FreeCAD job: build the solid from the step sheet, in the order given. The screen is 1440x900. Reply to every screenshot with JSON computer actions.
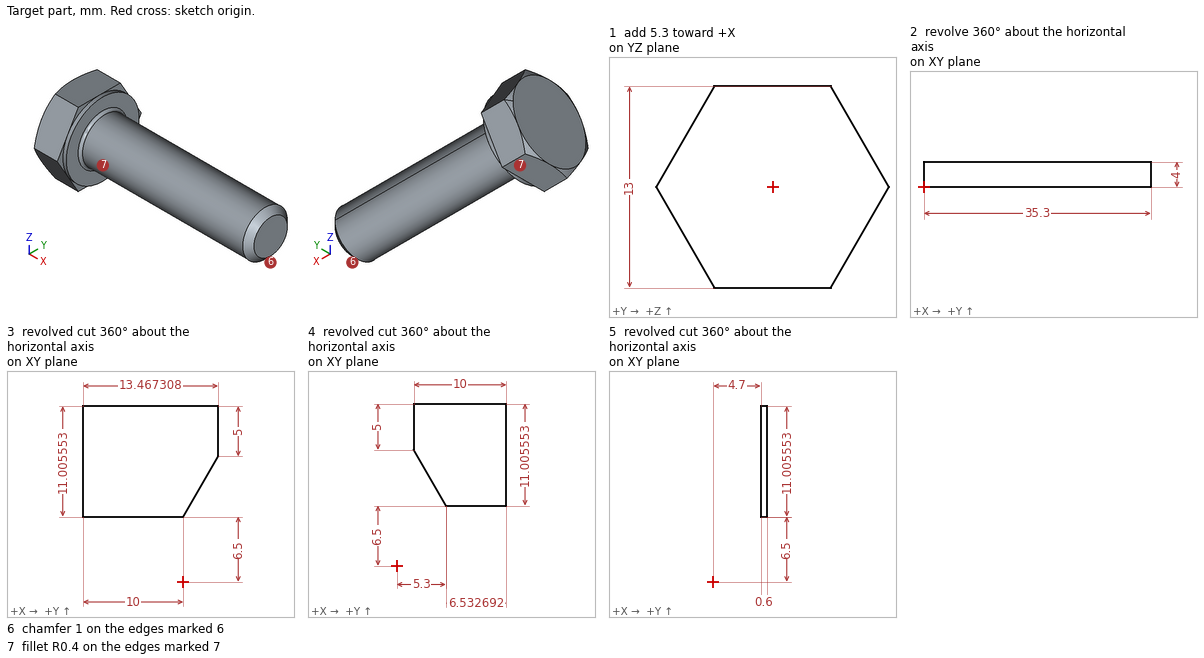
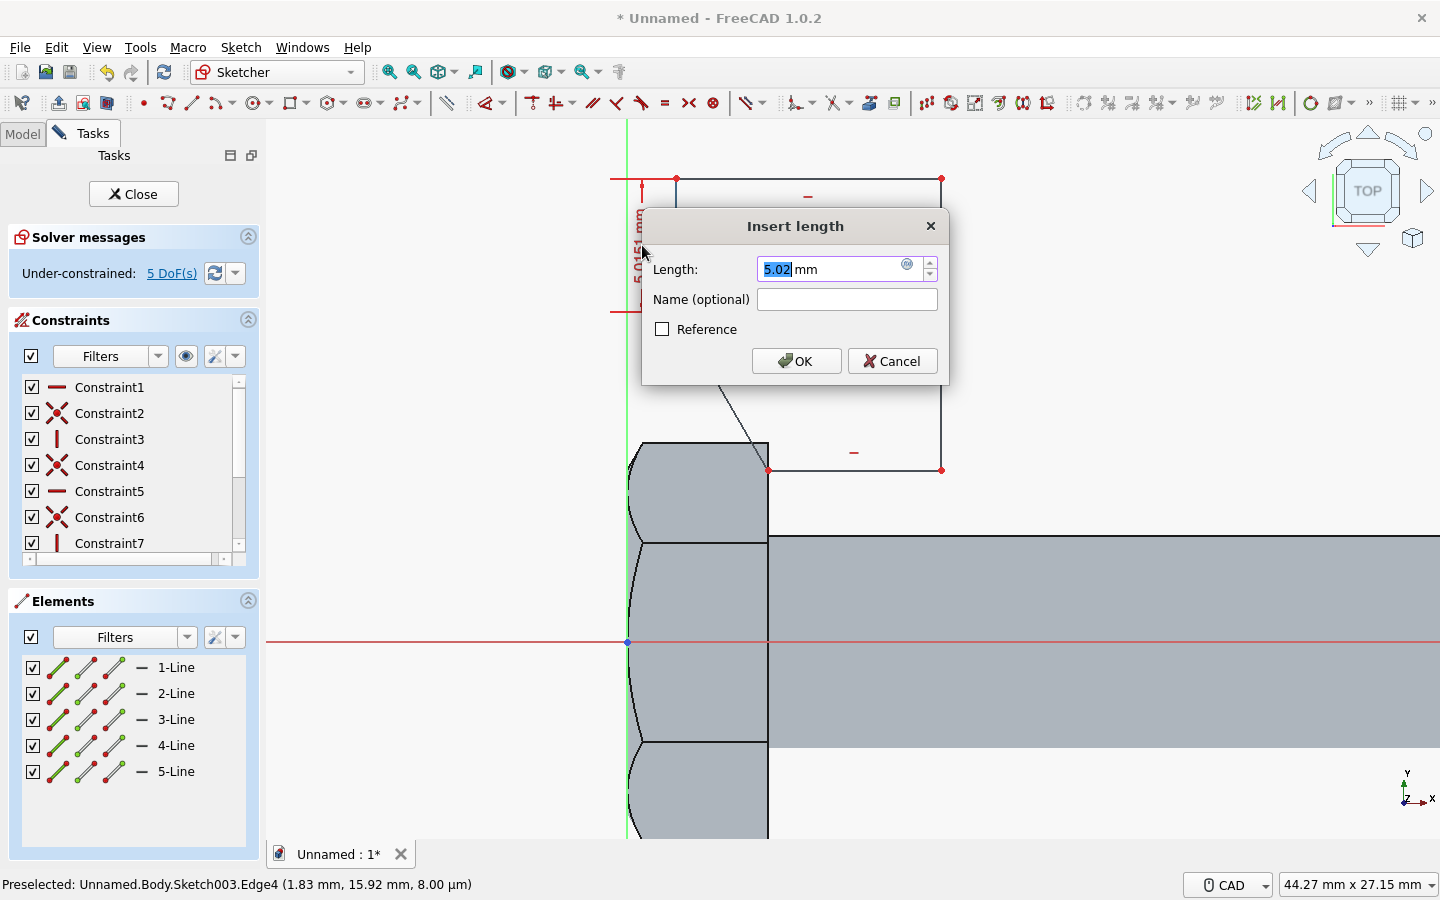
{"action": "type", "text": "5"}
{"action": "key", "text": "Return"}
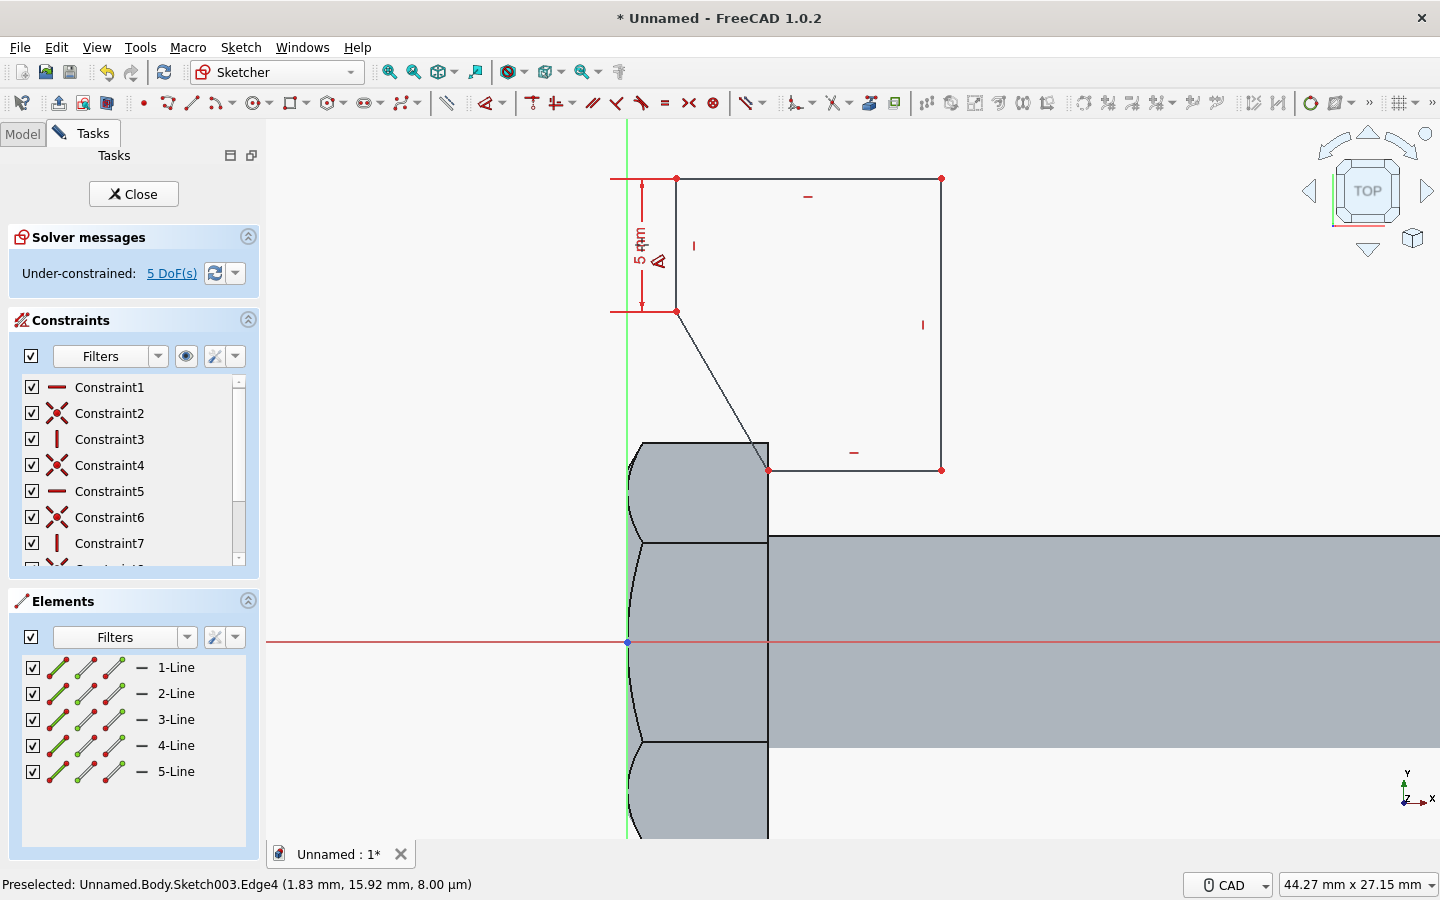
{"action": "left_click", "coordinate": [862, 179]}
{"action": "left_click", "coordinate": [809, 213]}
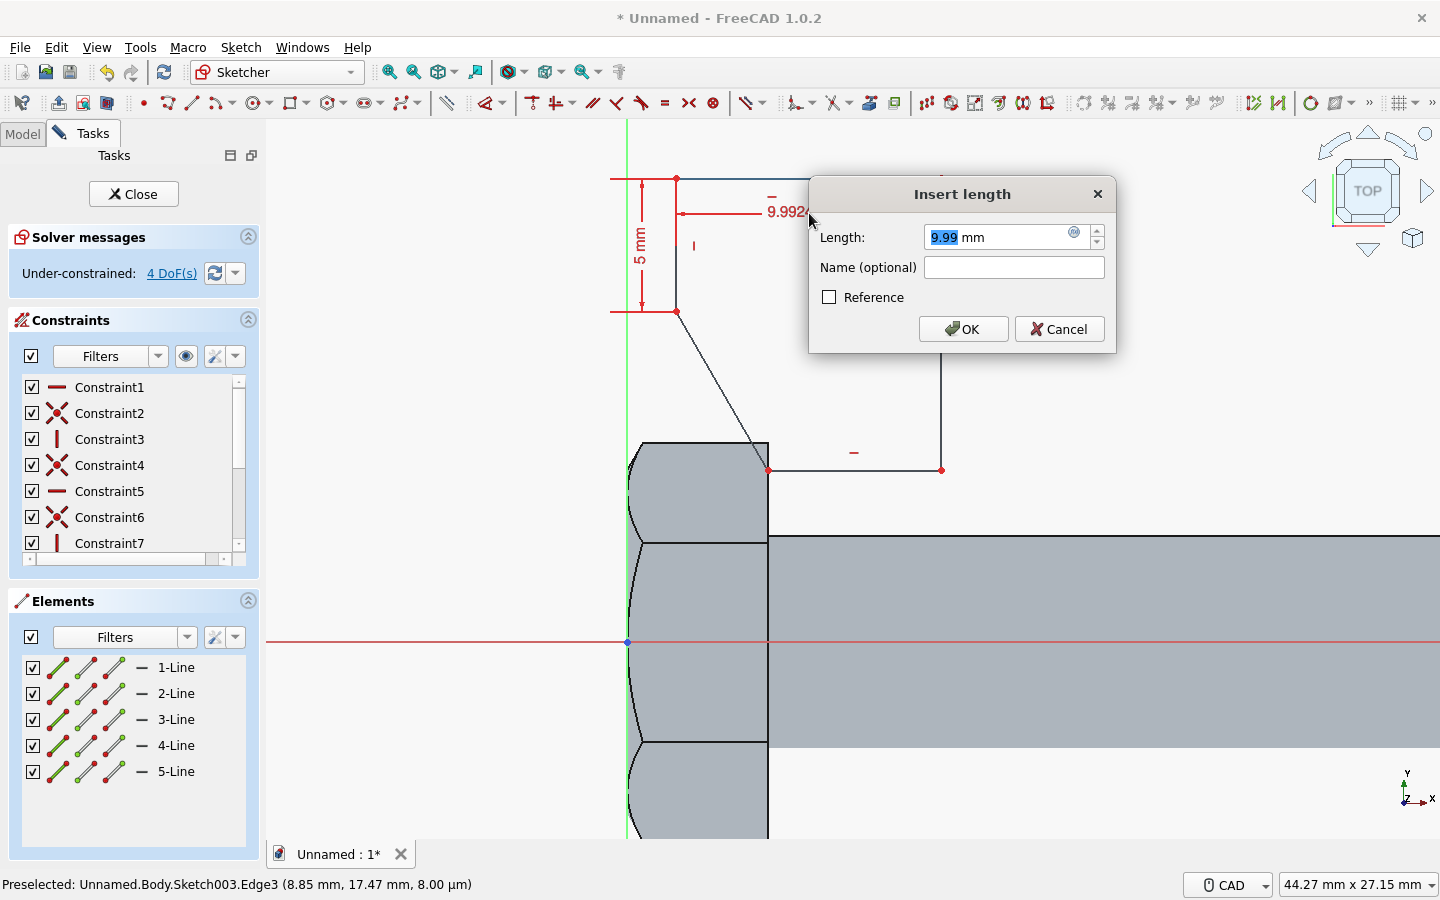
{"action": "type", "text": "10"}
{"action": "key", "text": "Return"}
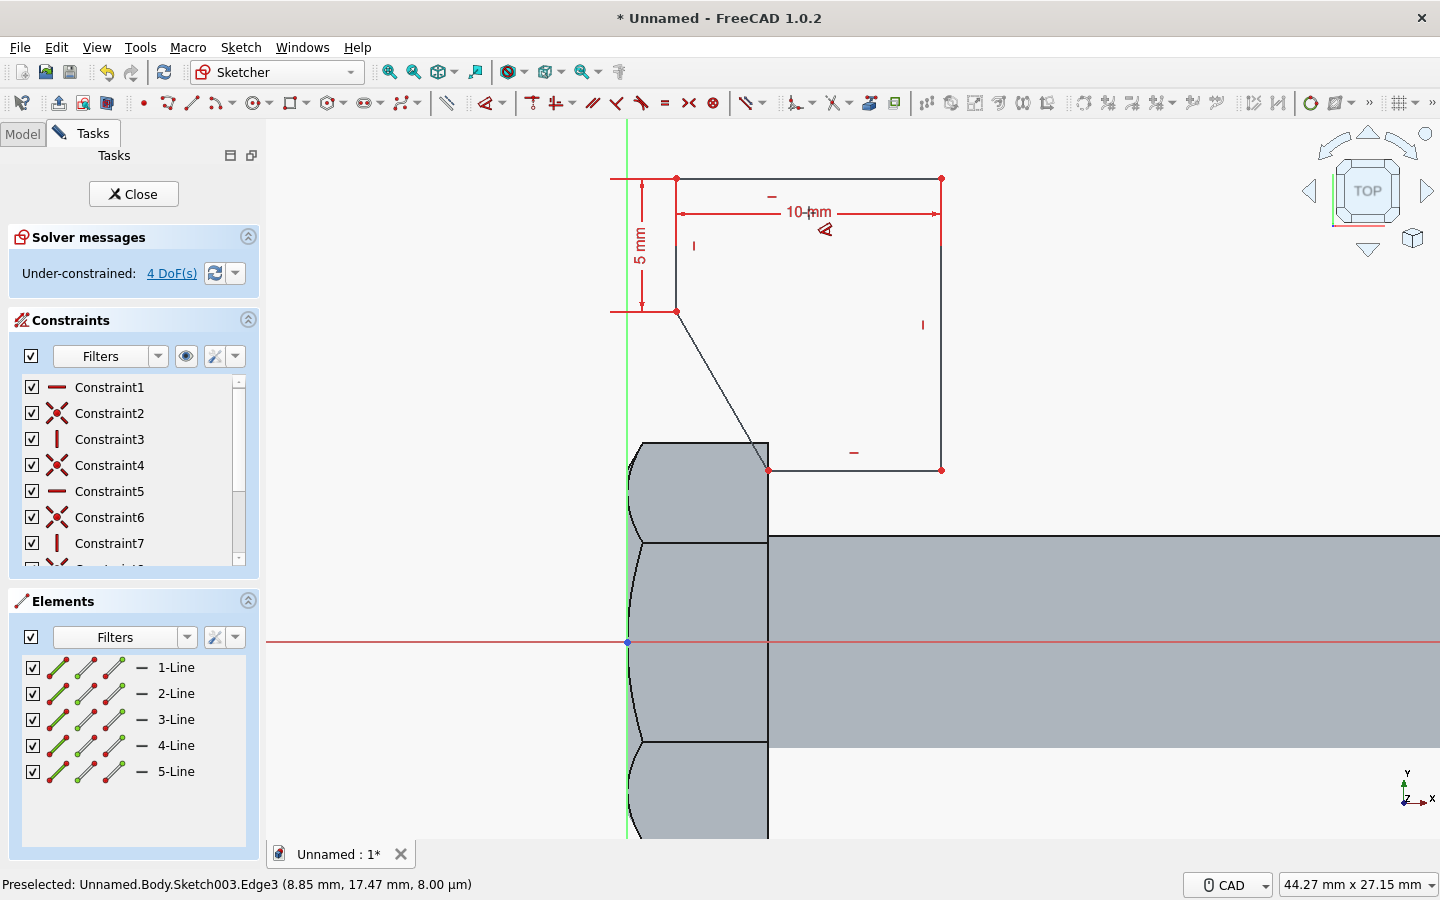
{"action": "left_click", "coordinate": [768, 471]}
{"action": "left_click", "coordinate": [698, 676]}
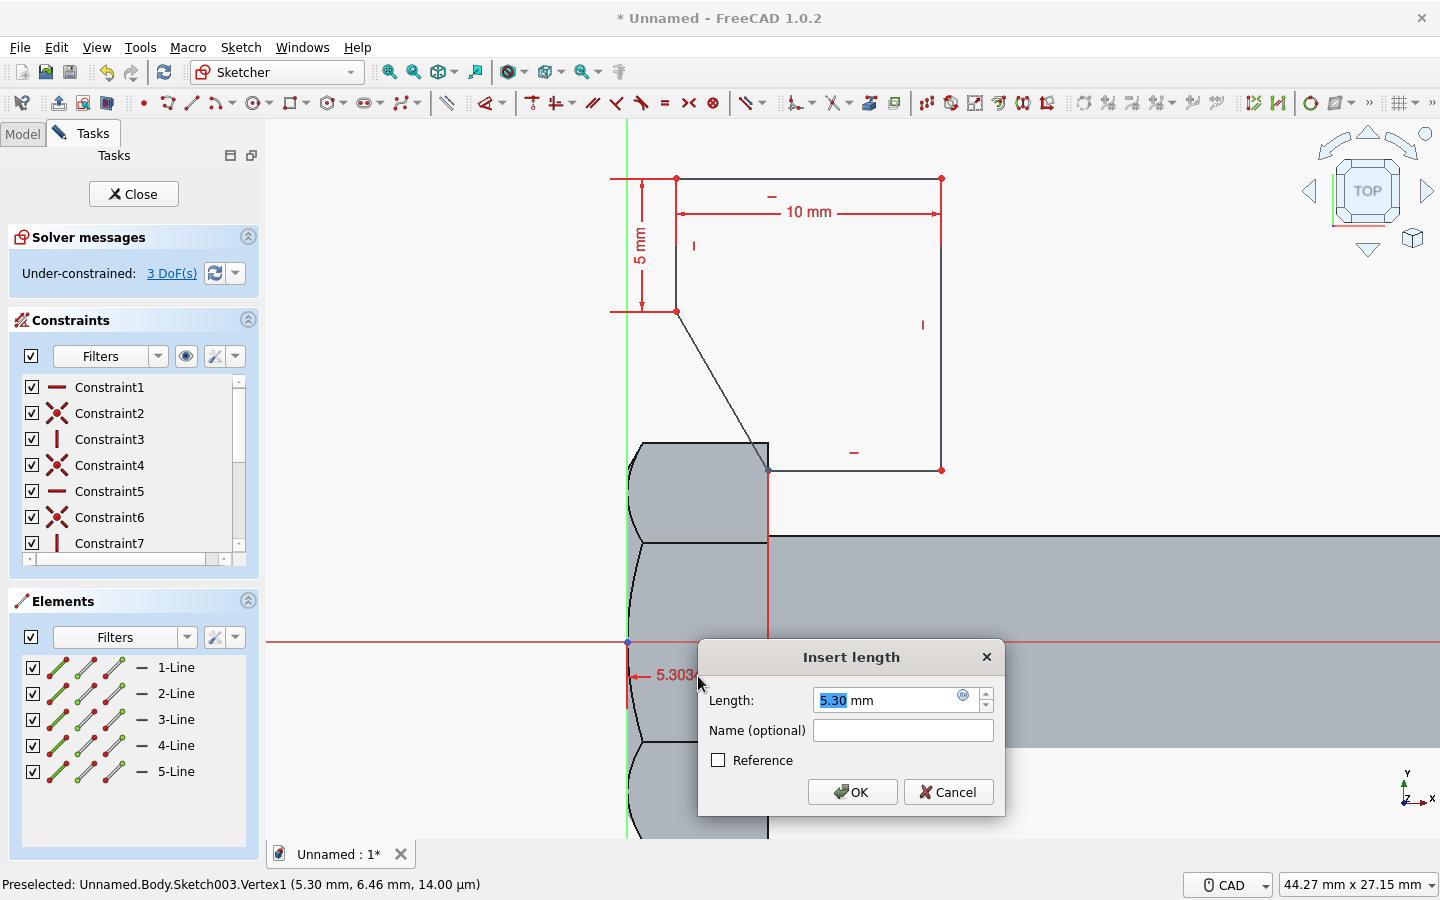
{"action": "type", "text": "5.3"}
{"action": "key", "text": "Return"}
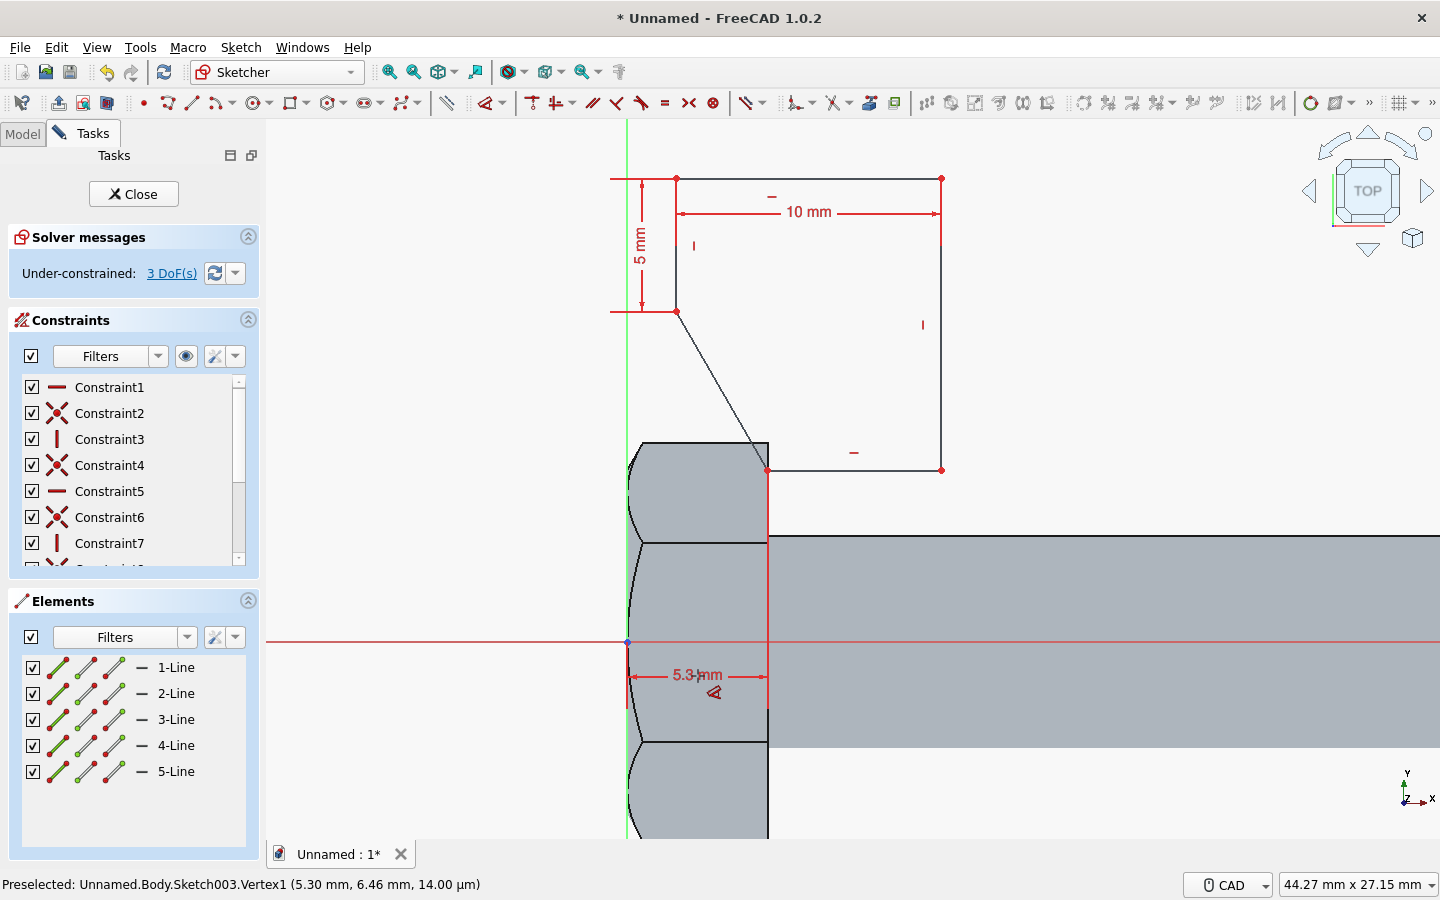
{"action": "left_click", "coordinate": [768, 471]}
{"action": "left_click", "coordinate": [593, 557]}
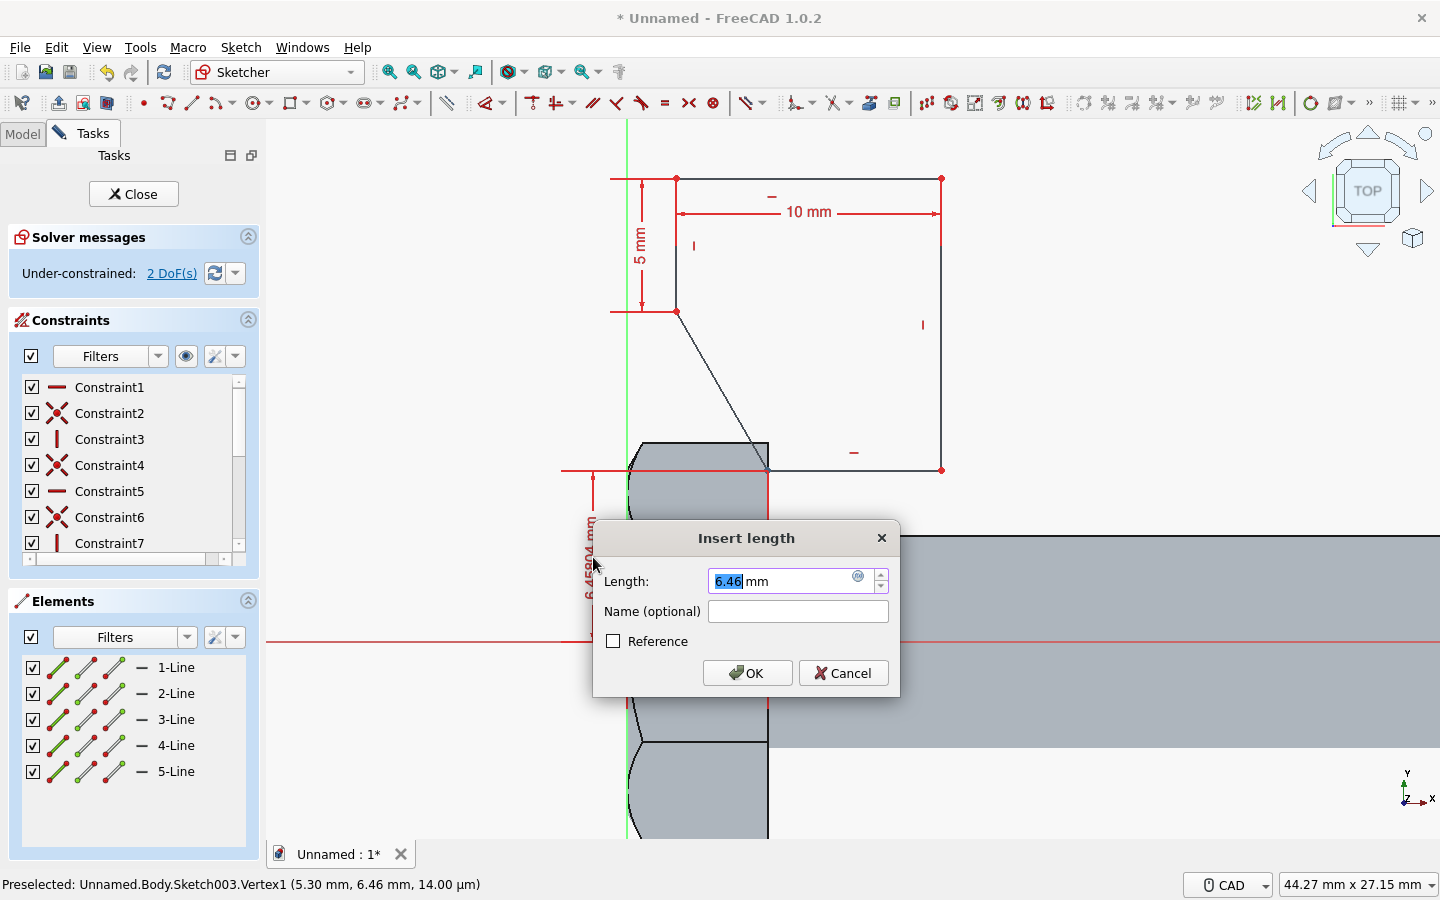
{"action": "type", "text": "6.5"}
{"action": "key", "text": "Return"}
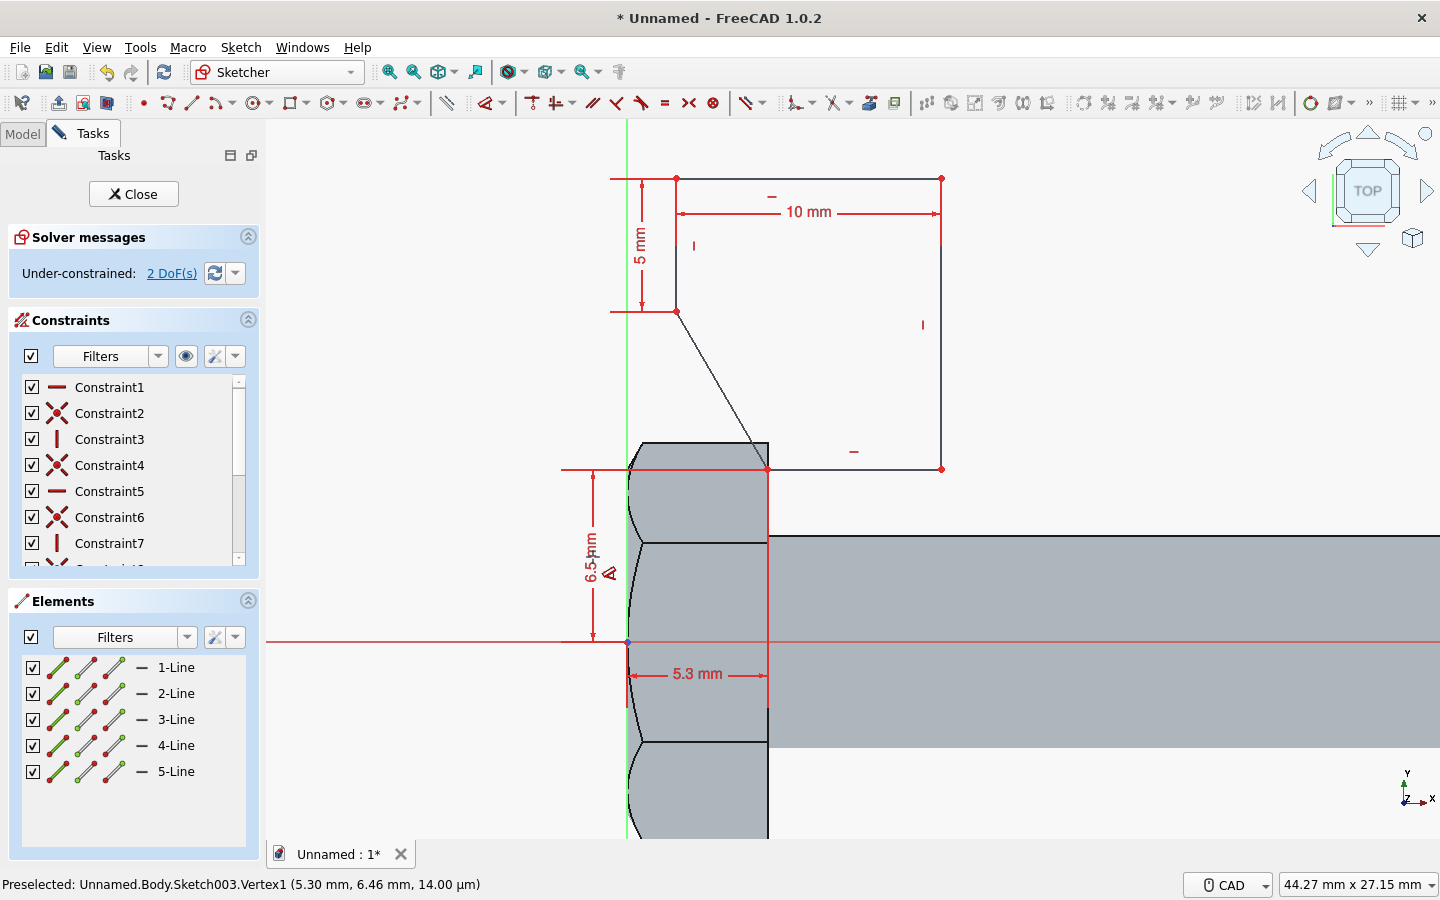
{"action": "left_click", "coordinate": [820, 470]}
{"action": "left_click", "coordinate": [855, 504]}